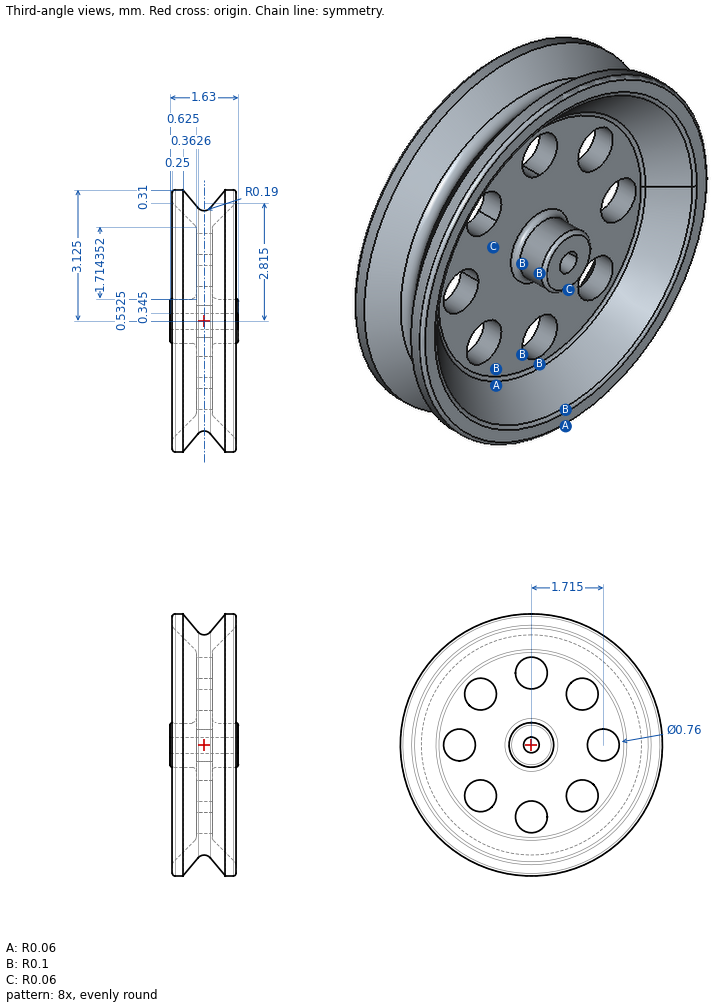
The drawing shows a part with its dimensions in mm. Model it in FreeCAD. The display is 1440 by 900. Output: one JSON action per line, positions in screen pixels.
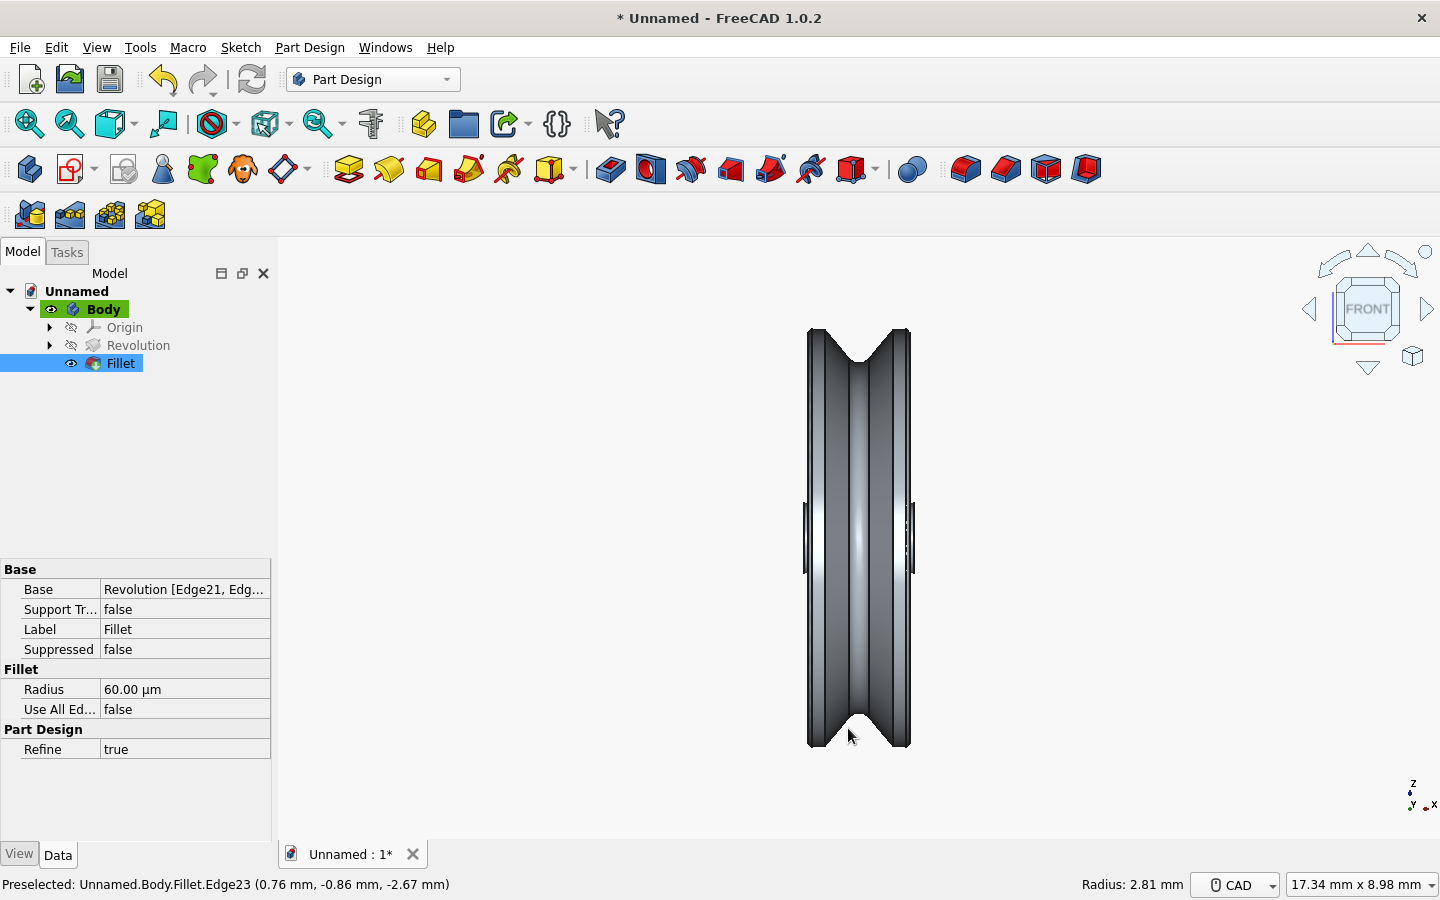
{"action": "key", "text": "3"}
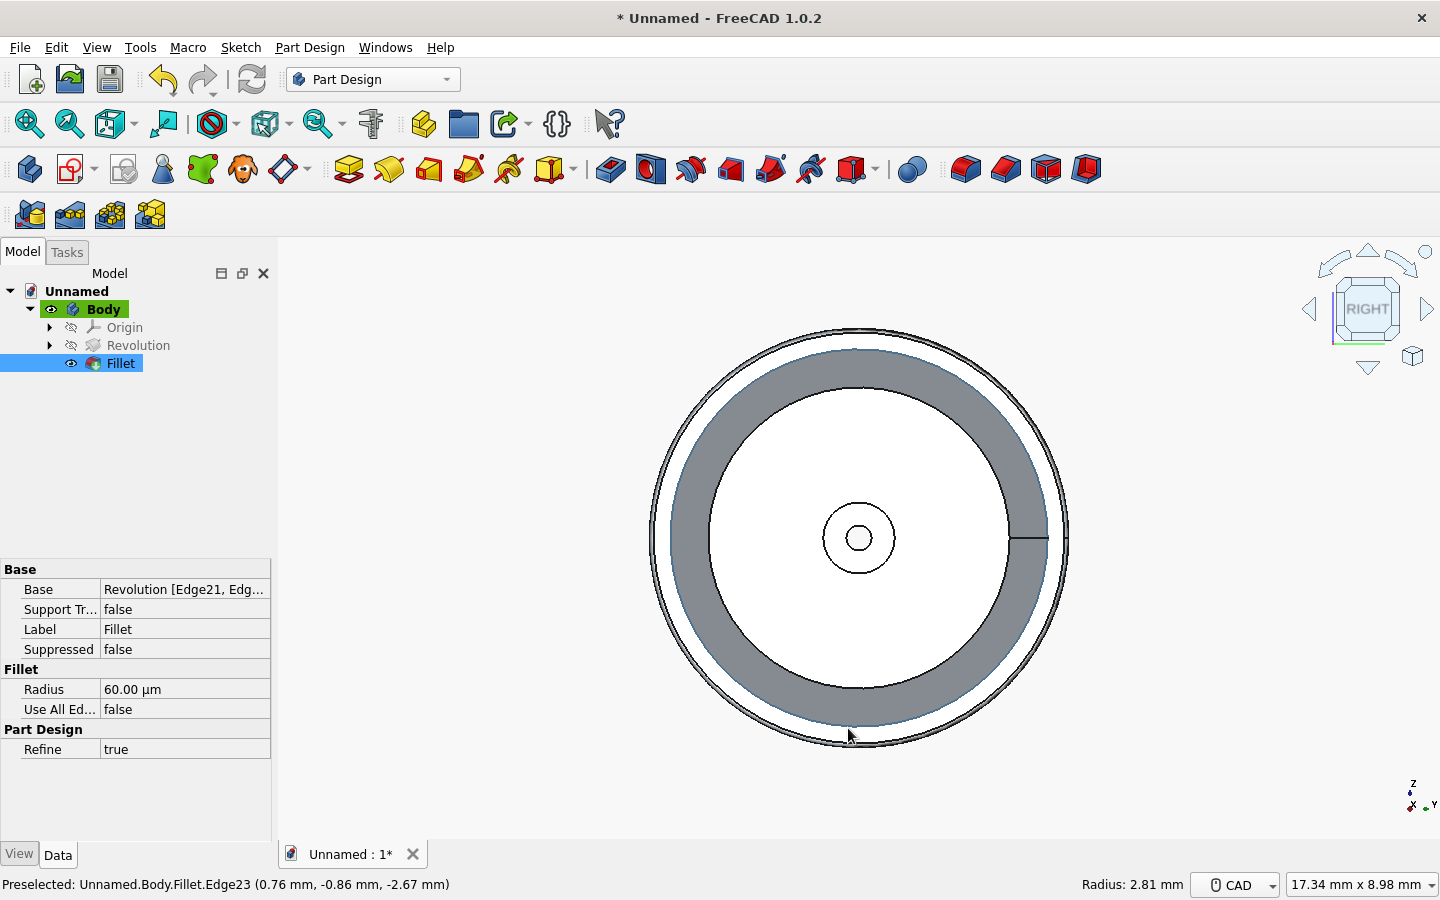
{"action": "key", "text": "5"}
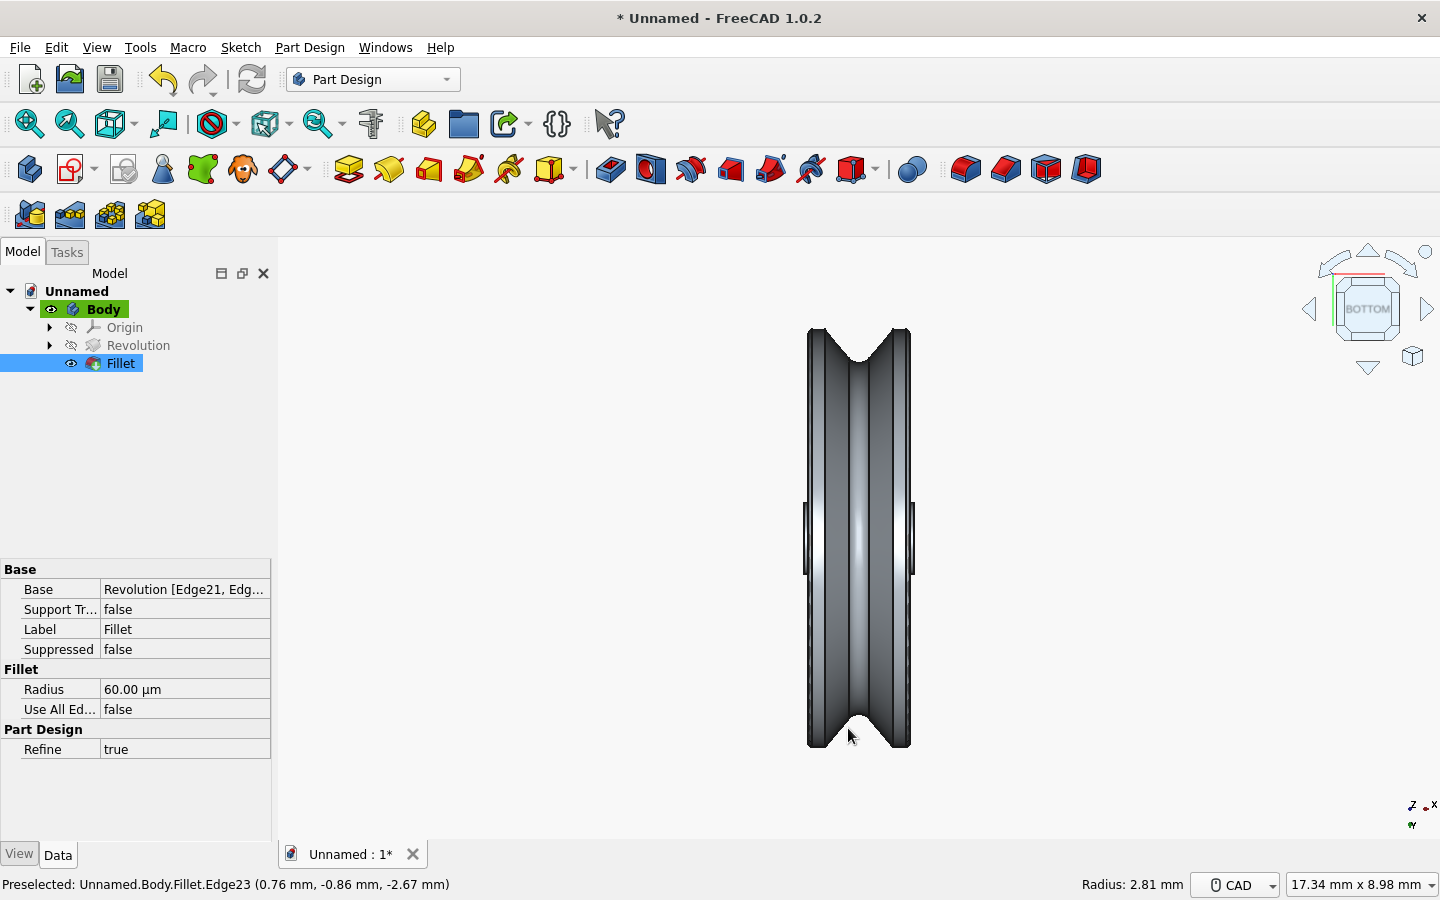
{"action": "key", "text": "4"}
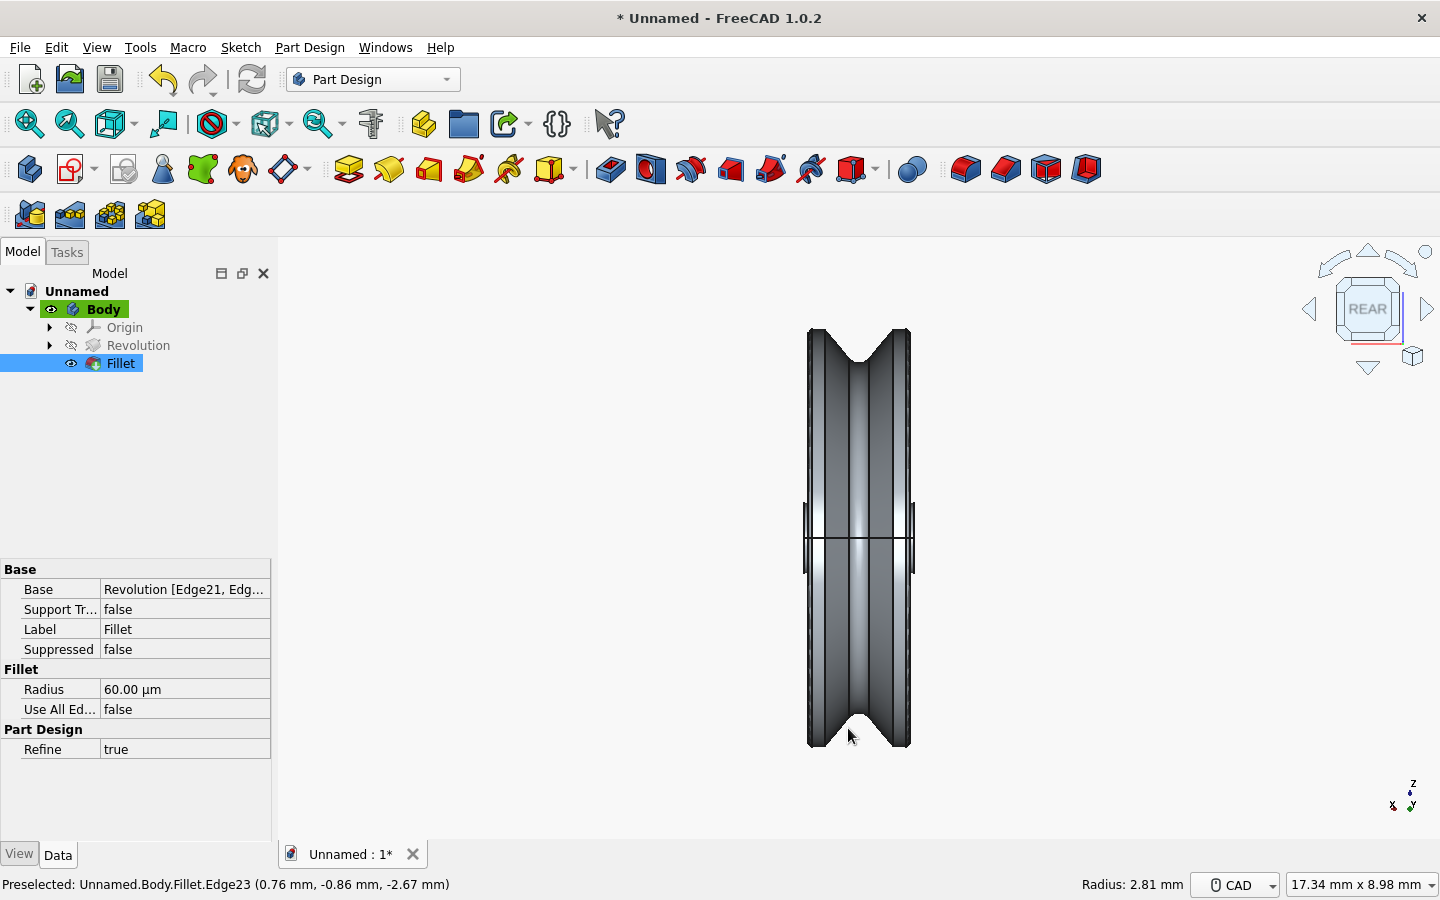
{"action": "key", "text": "6"}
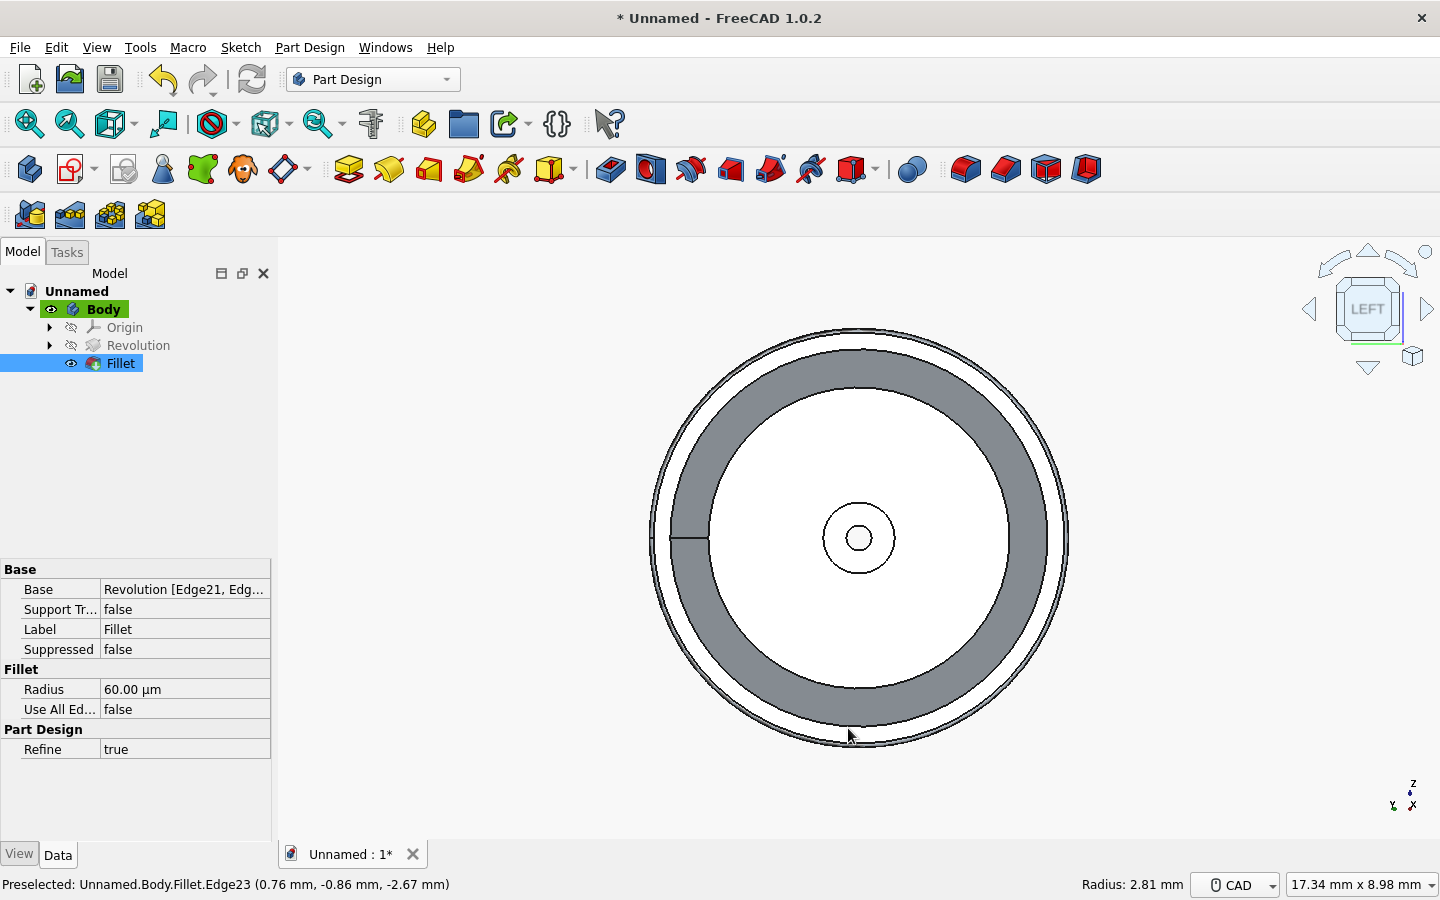
{"action": "left_click", "coordinate": [1048, 537], "text": "ctrl"}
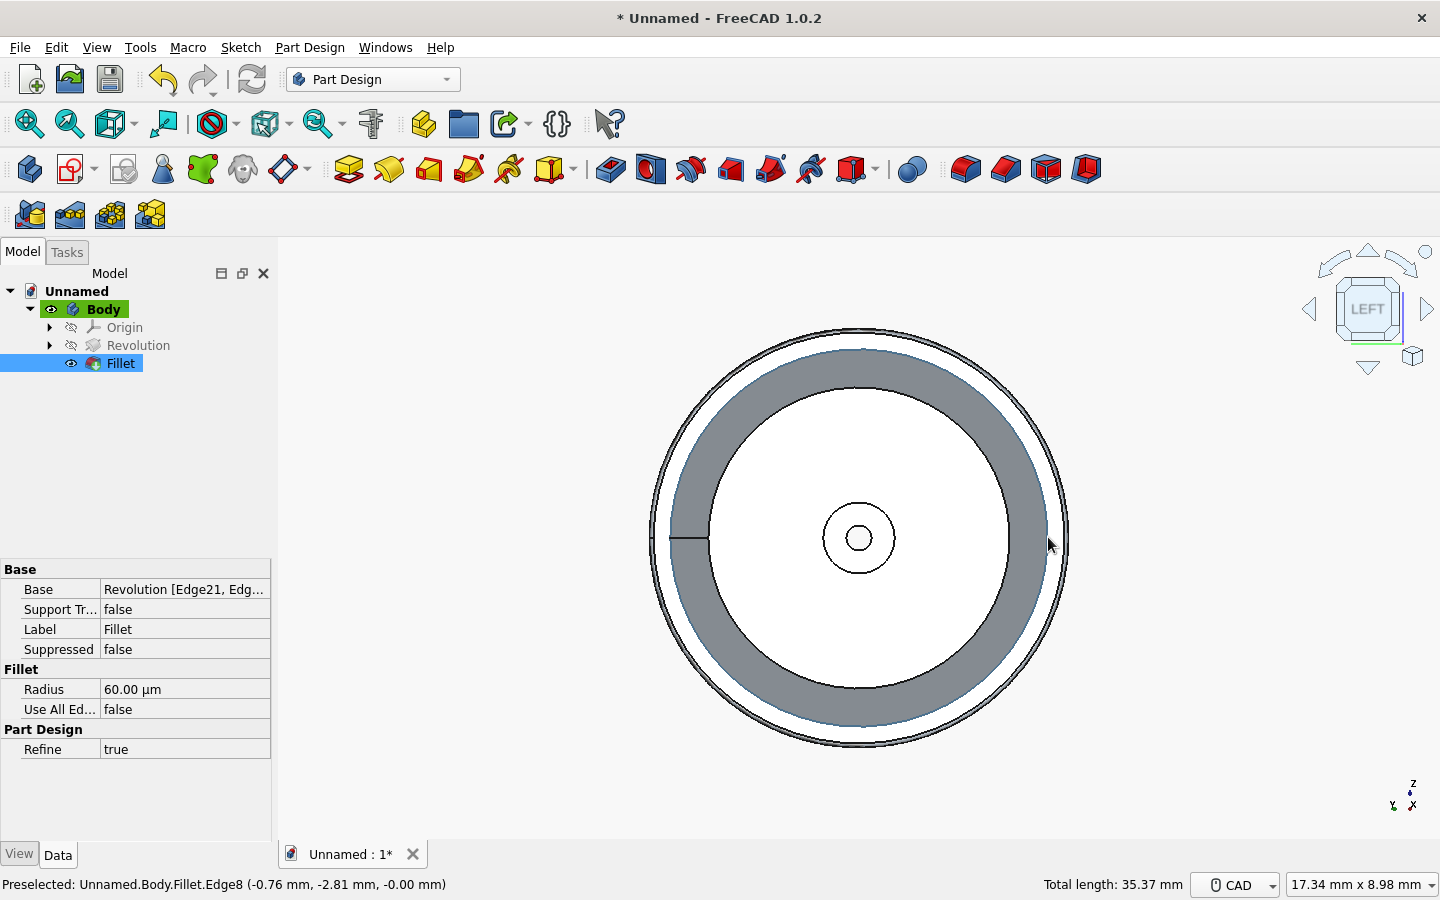
{"action": "key", "text": "v 3"}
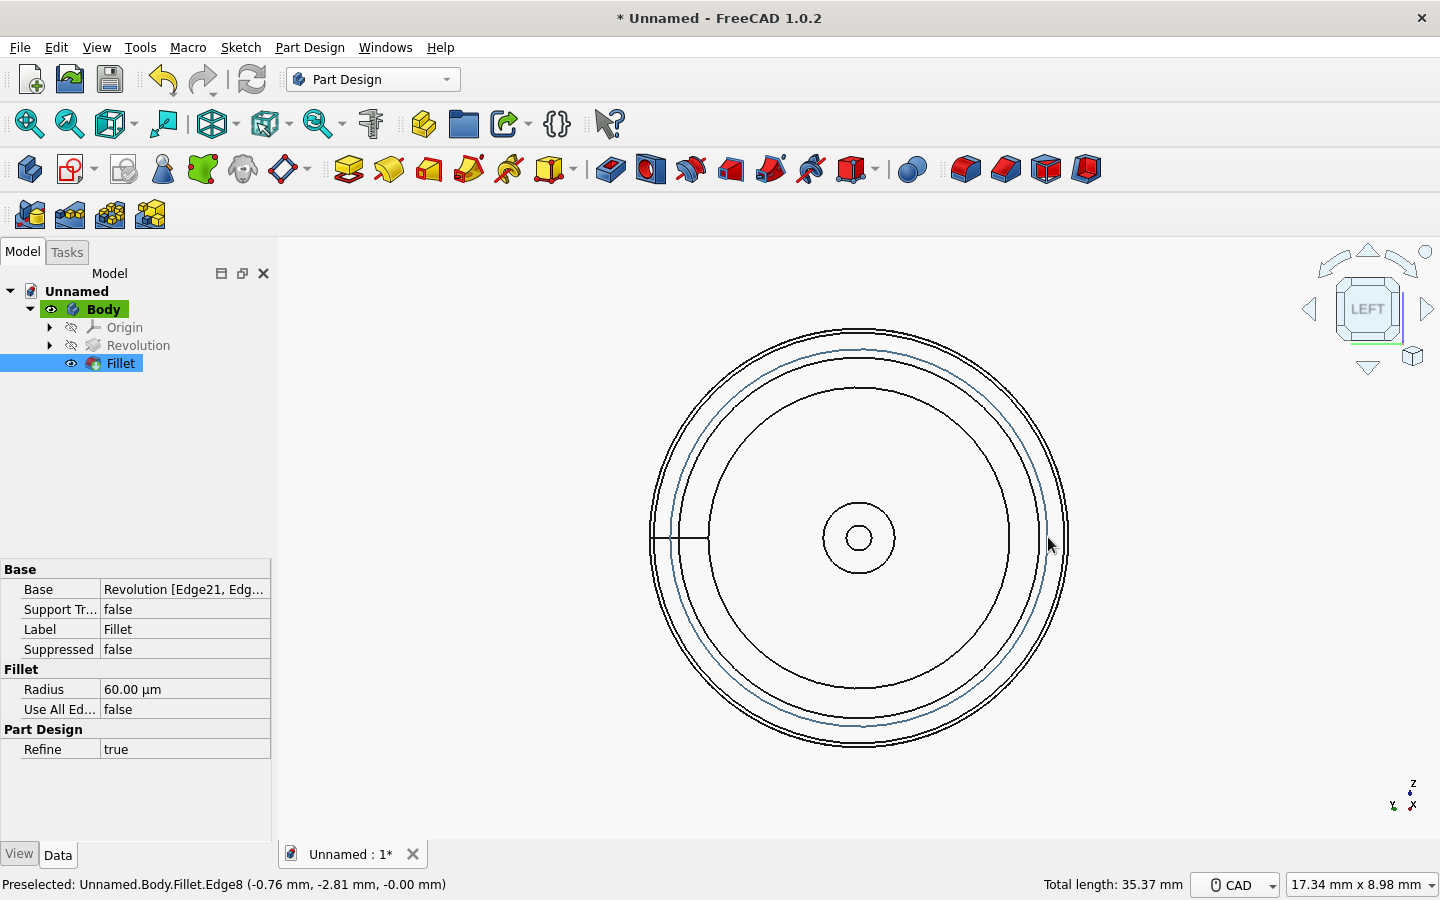
{"action": "key", "text": "0"}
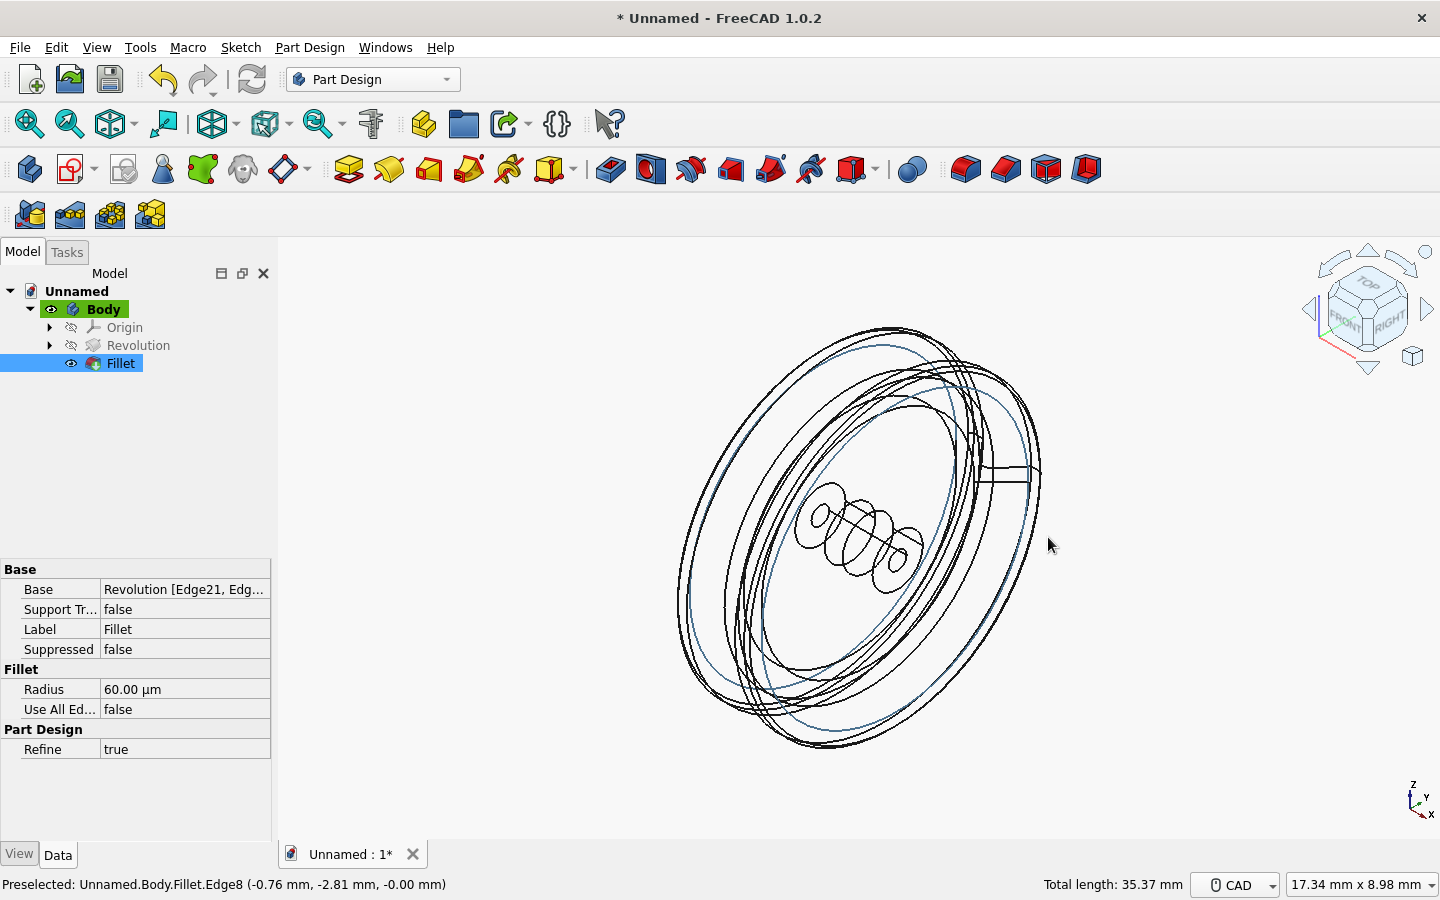
{"action": "left_click", "coordinate": [825, 546], "text": "ctrl"}